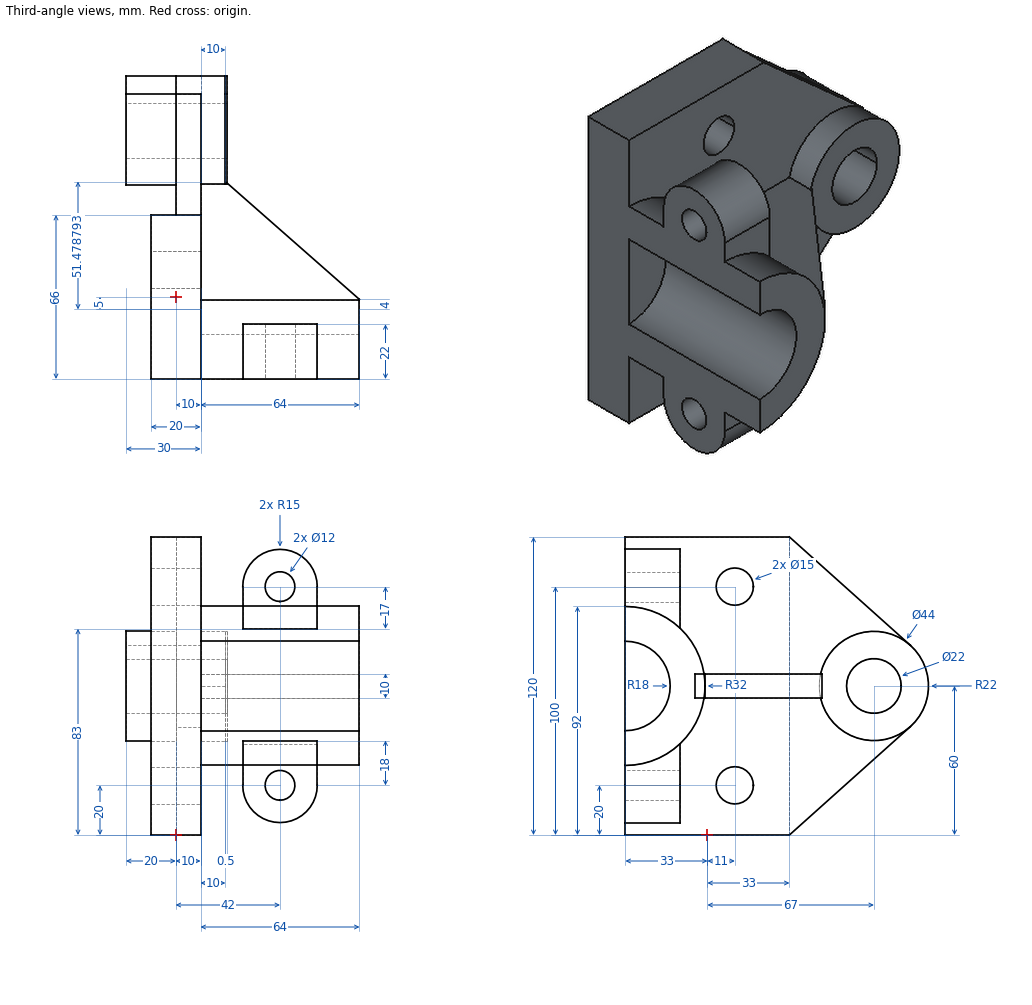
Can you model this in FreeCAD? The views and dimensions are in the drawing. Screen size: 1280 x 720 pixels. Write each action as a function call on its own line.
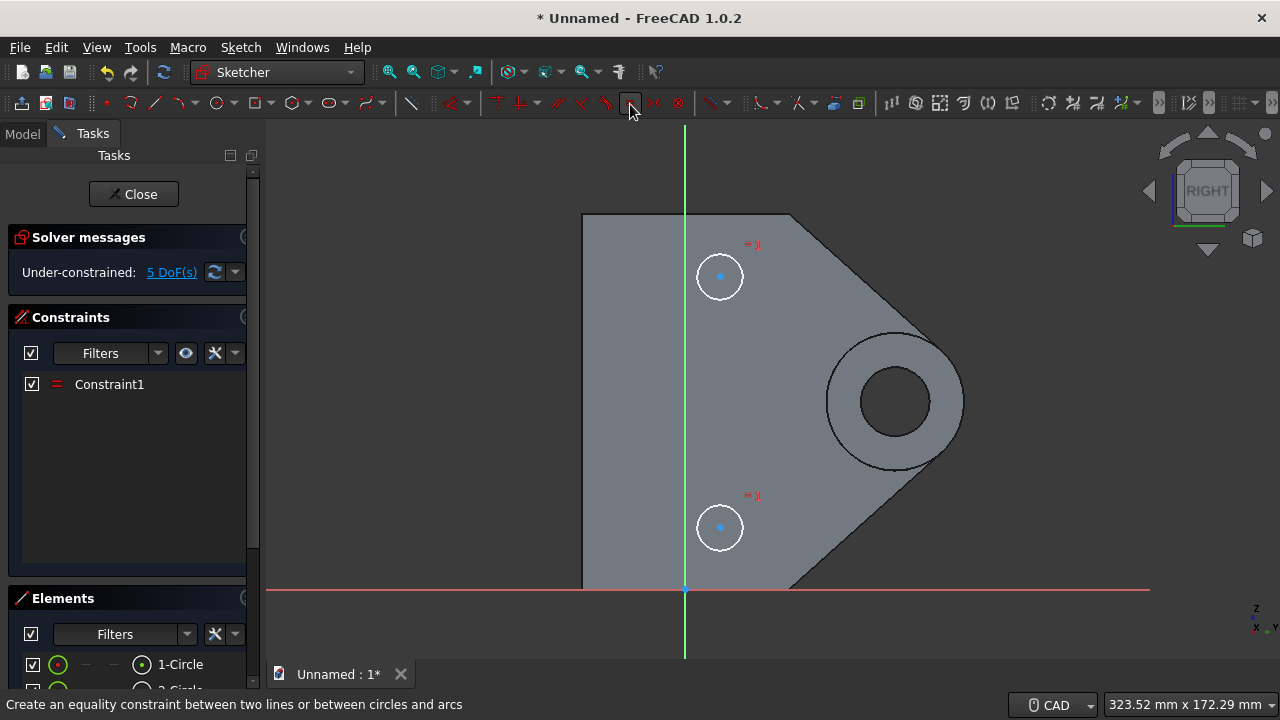
click(450, 104)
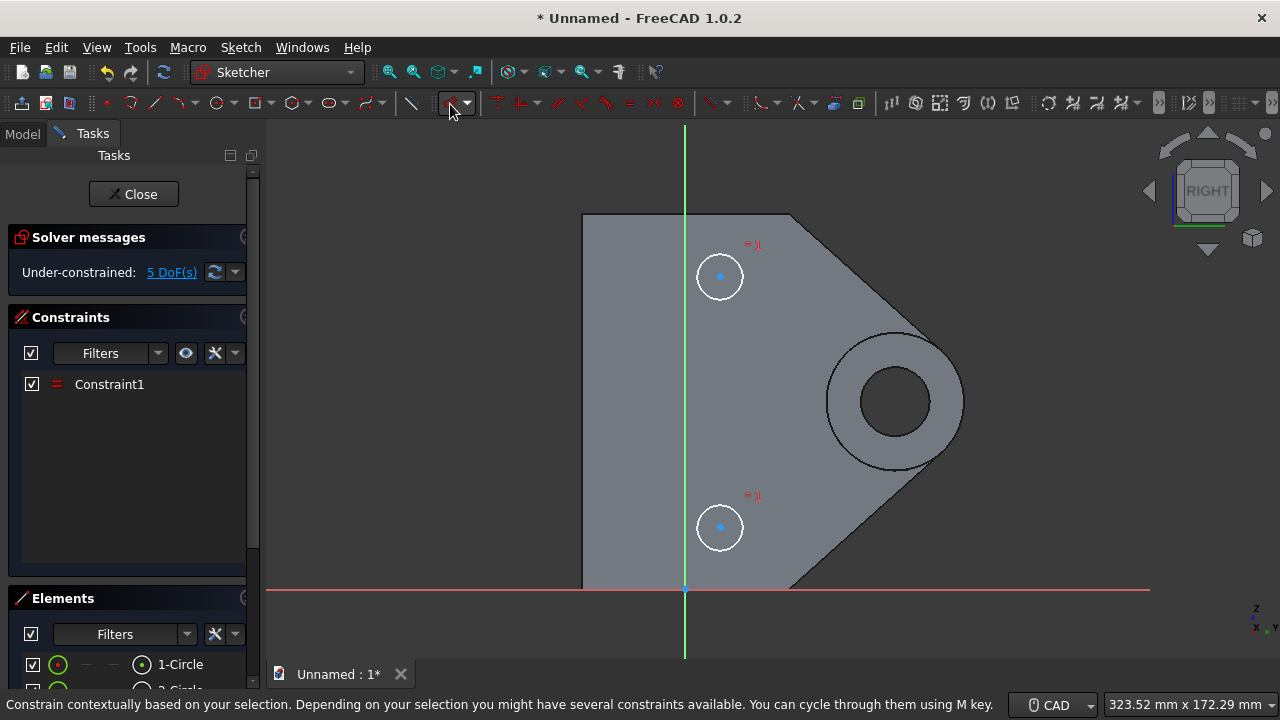
click(736, 261)
click(759, 238)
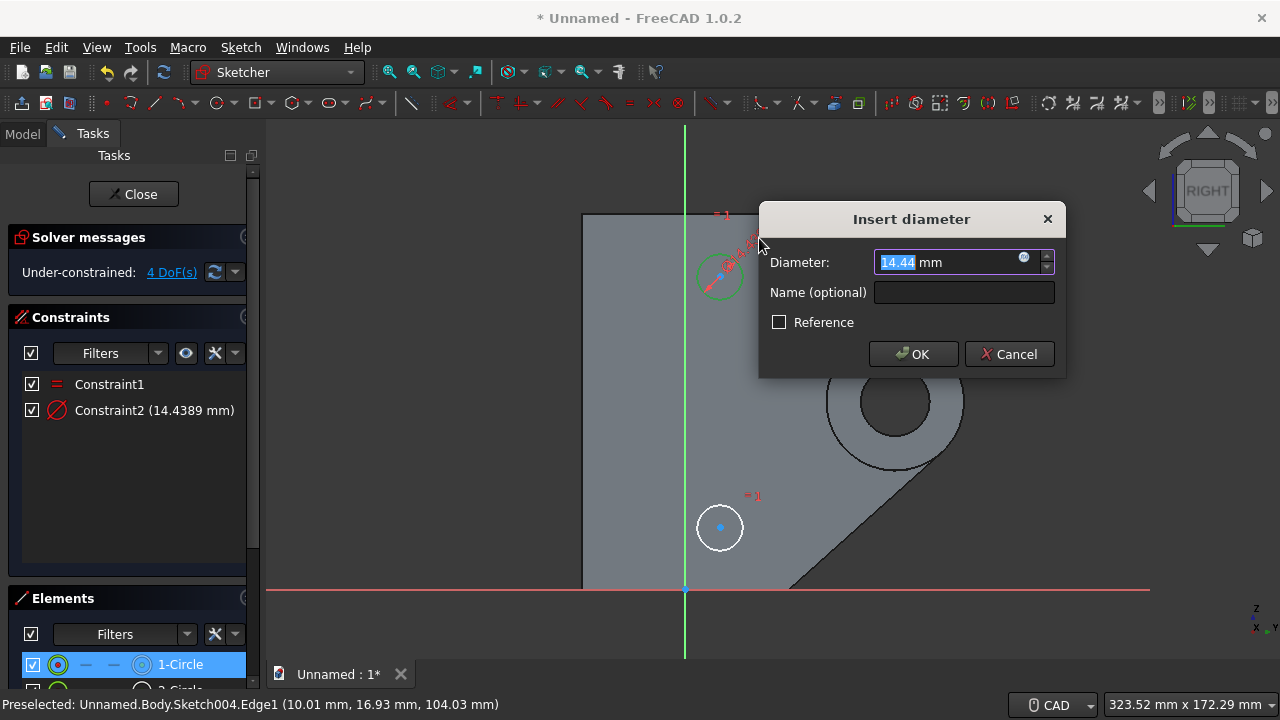
text(15)
key(Return)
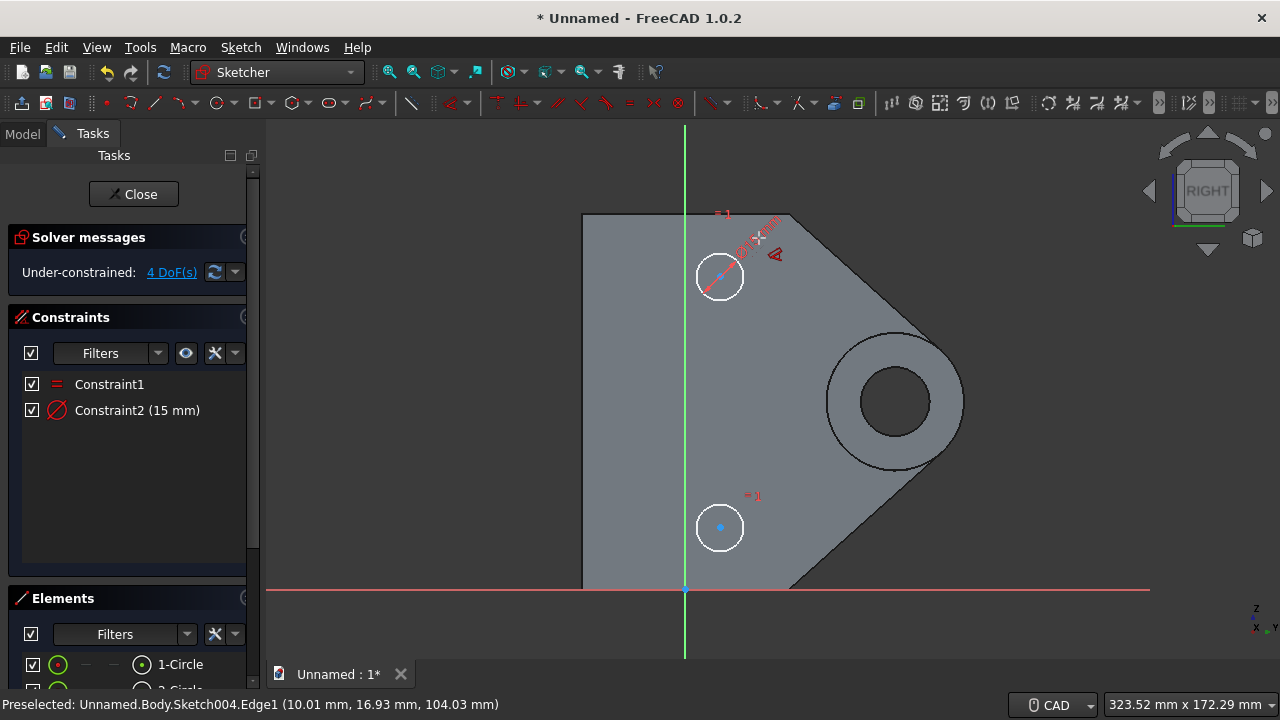
click(720, 277)
click(703, 624)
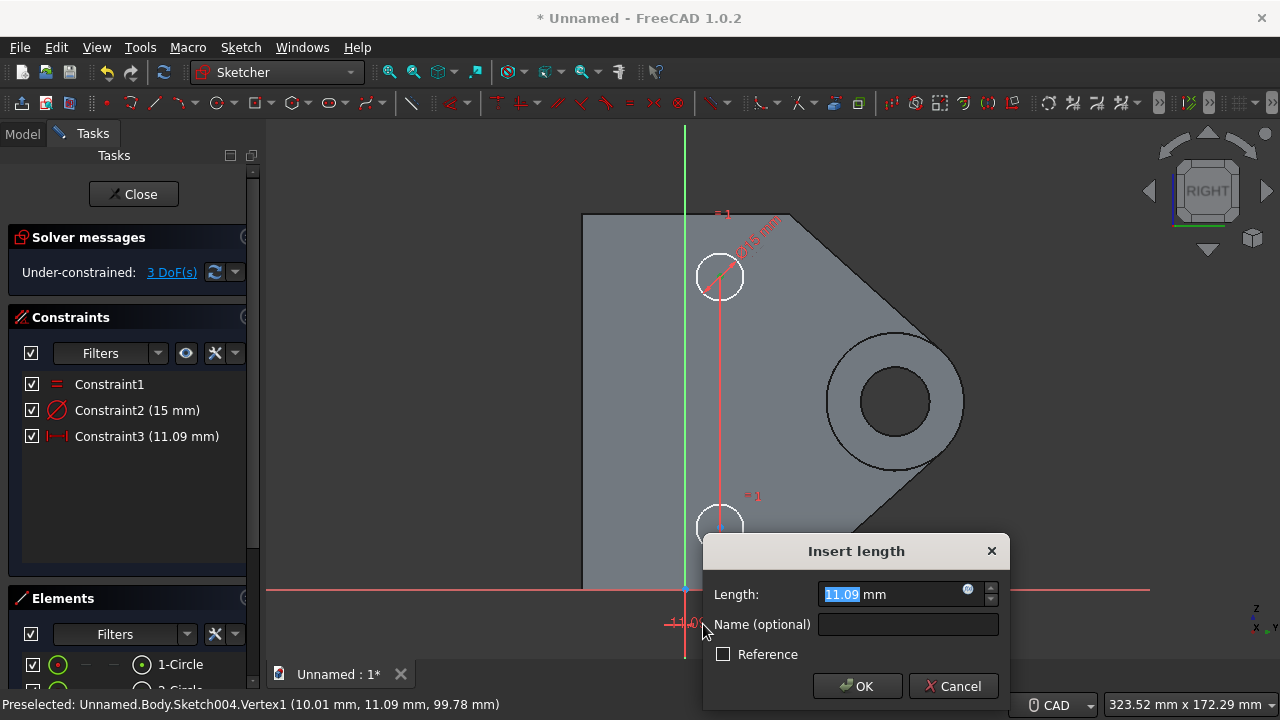
text(11)
key(Return)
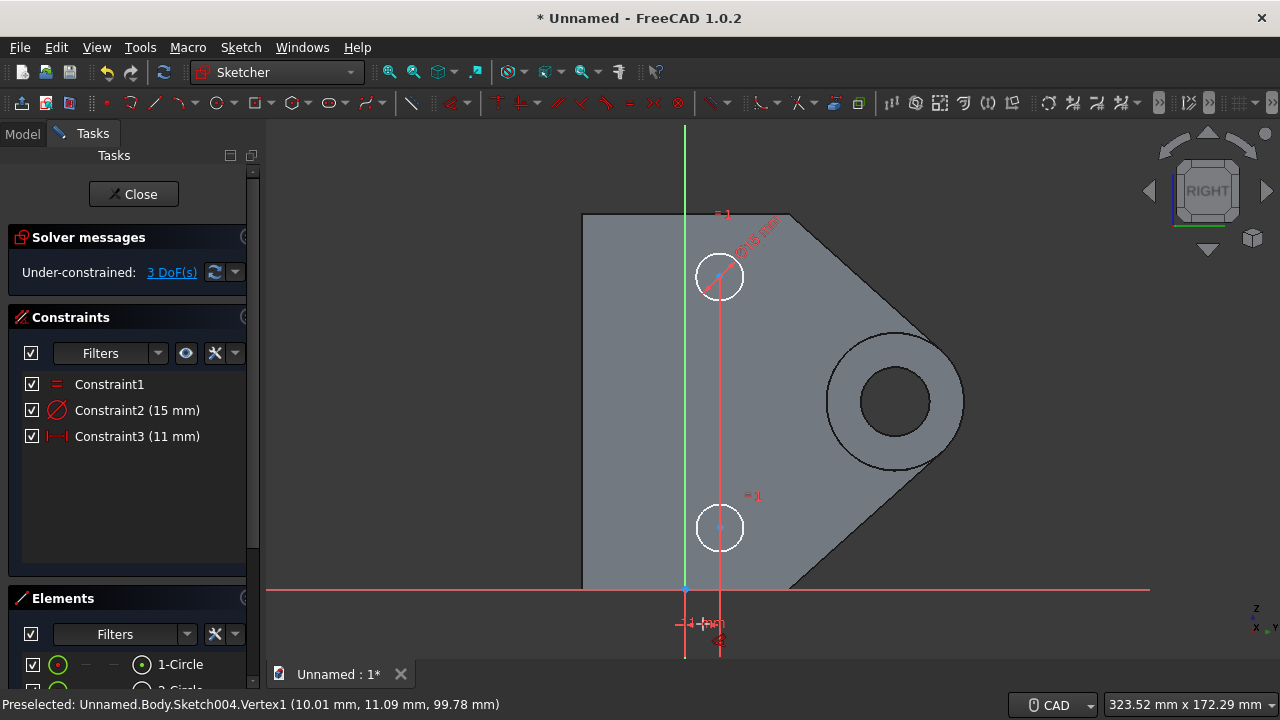
click(720, 528)
click(703, 494)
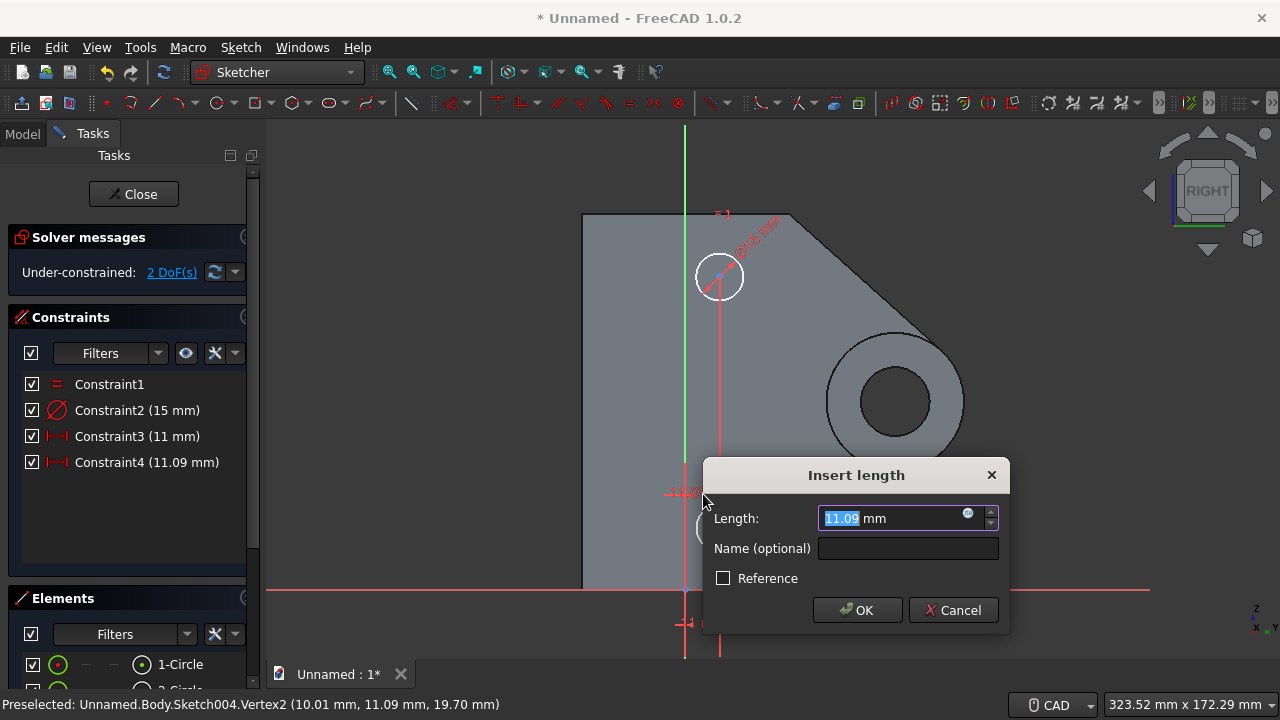
text(11)
key(Return)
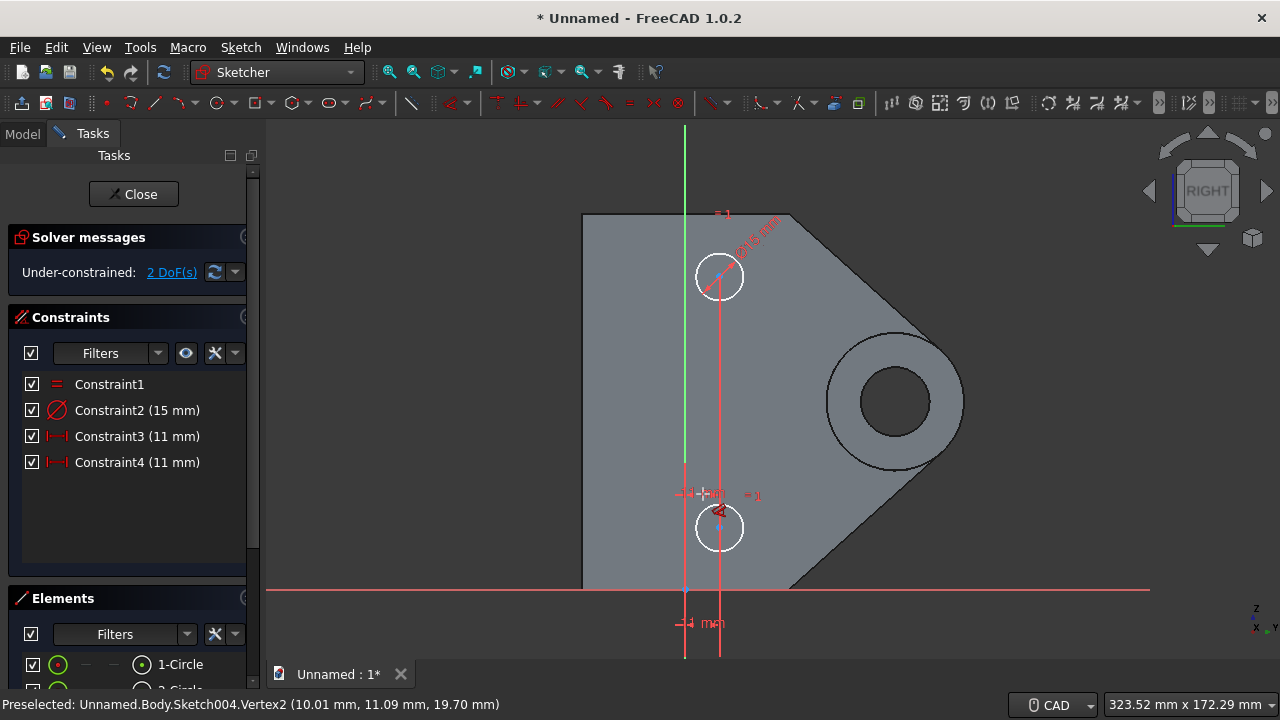
click(720, 528)
click(651, 559)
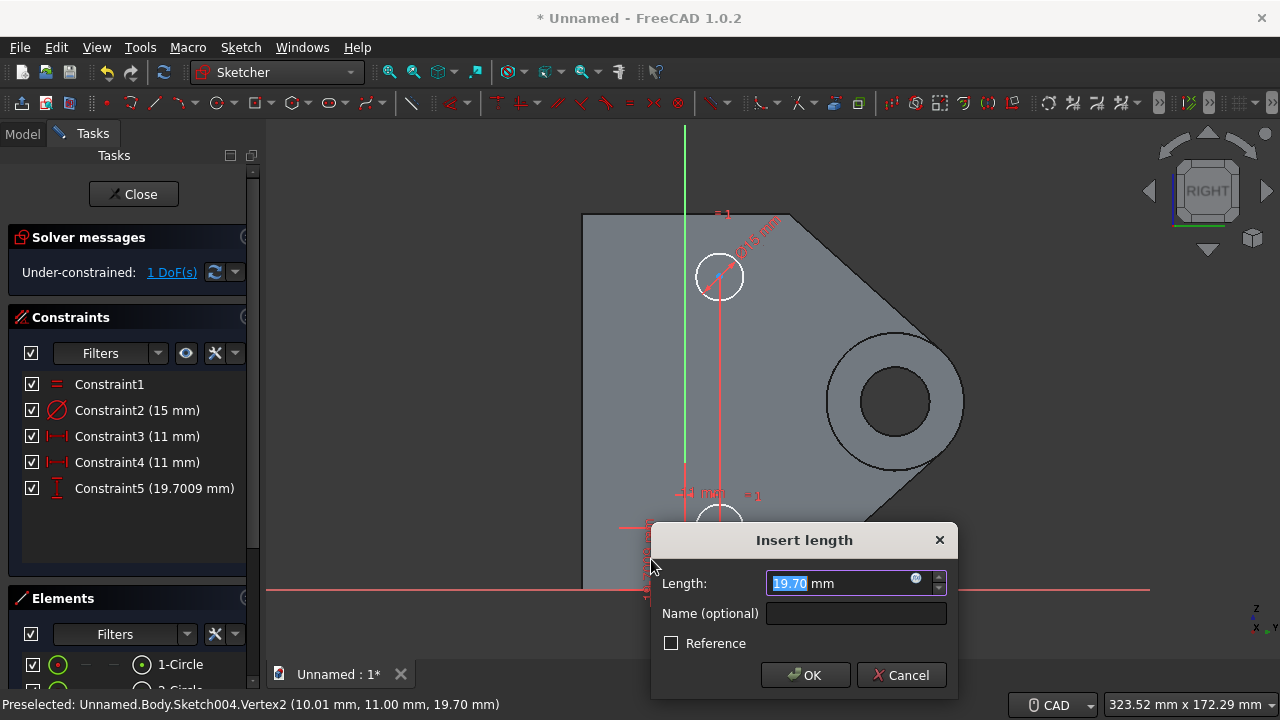
text(20)
key(Return)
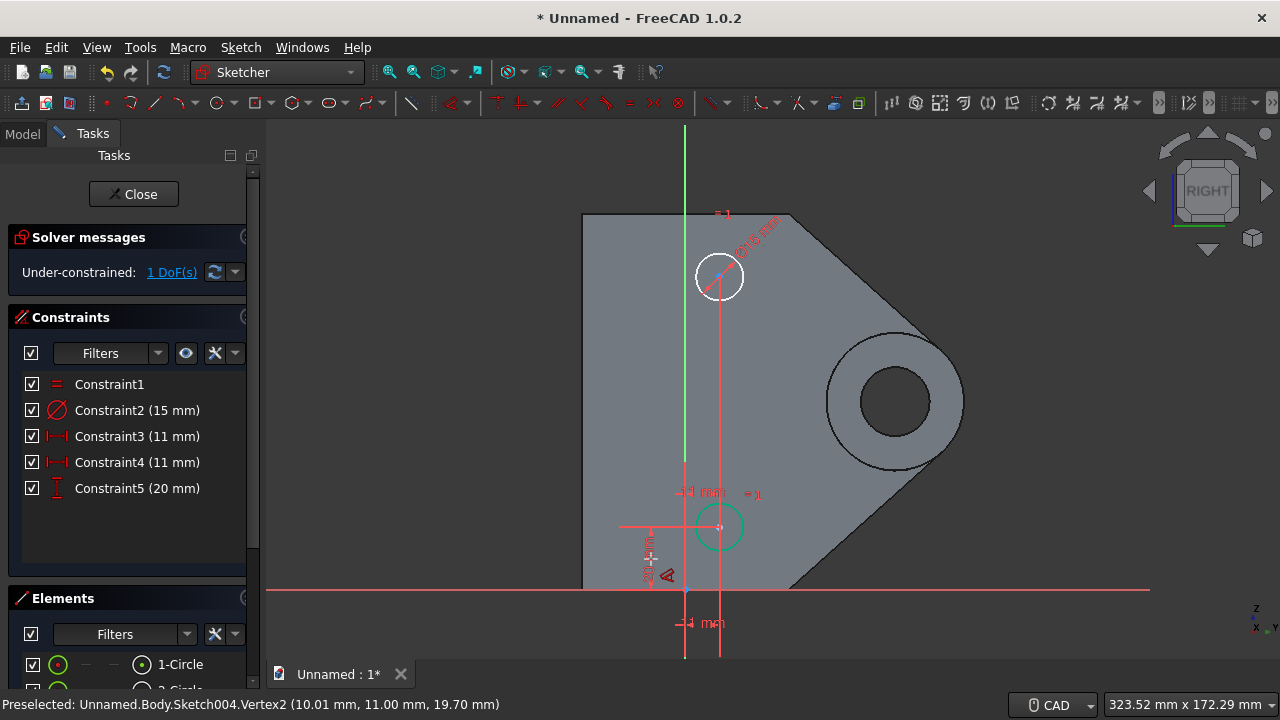
click(720, 277)
click(651, 433)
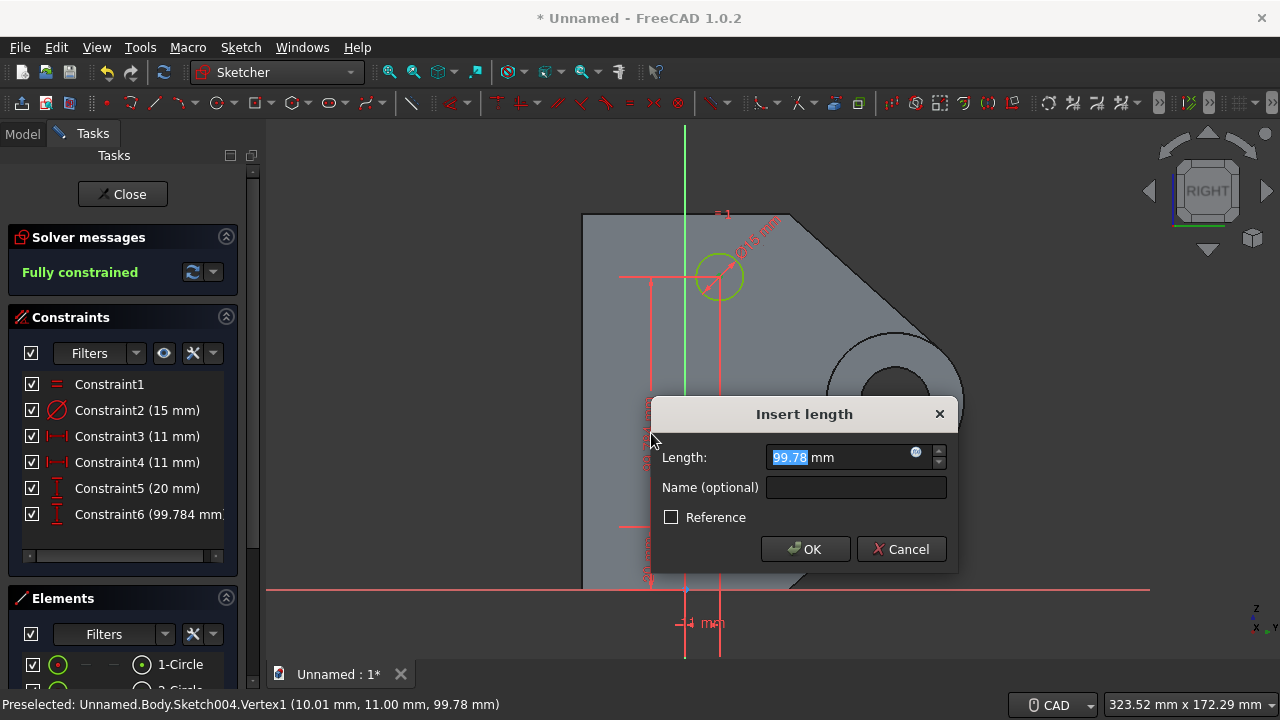
text(100)
key(Return)
key(Escape)